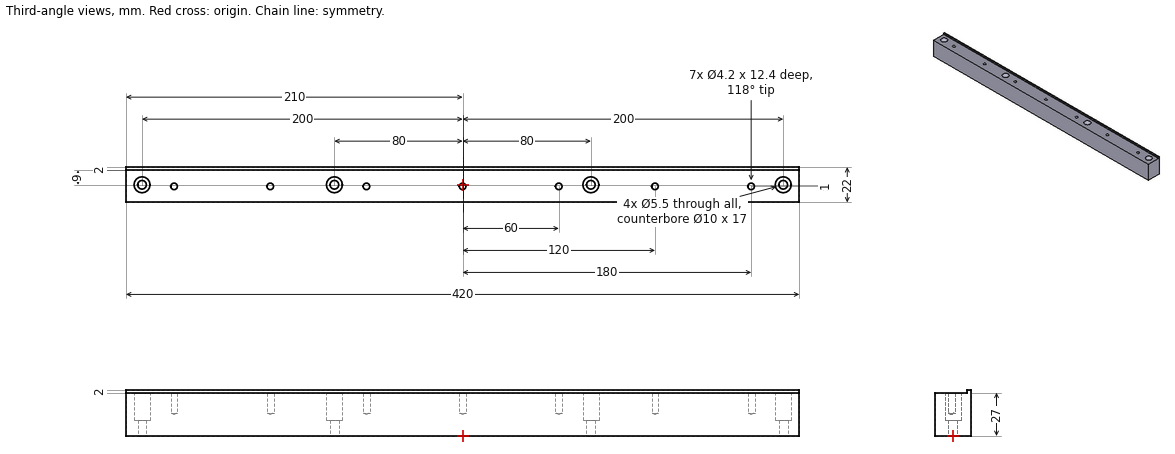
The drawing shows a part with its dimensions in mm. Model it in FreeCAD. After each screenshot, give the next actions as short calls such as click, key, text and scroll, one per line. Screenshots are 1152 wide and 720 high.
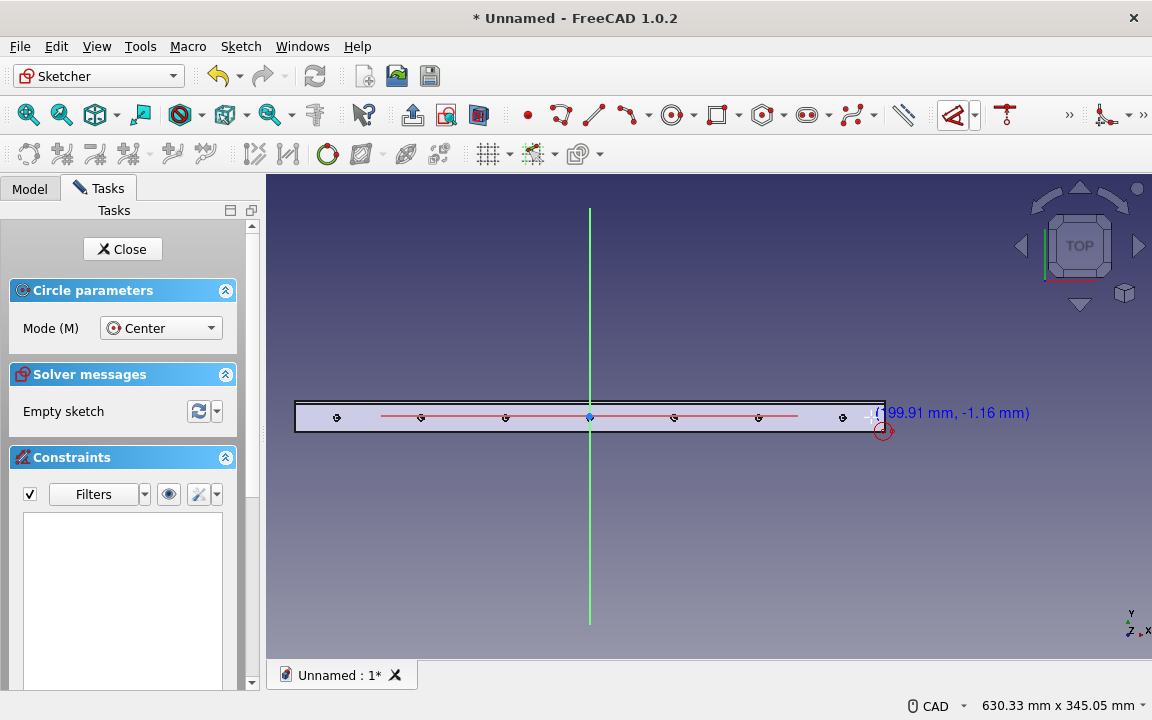
click(871, 417)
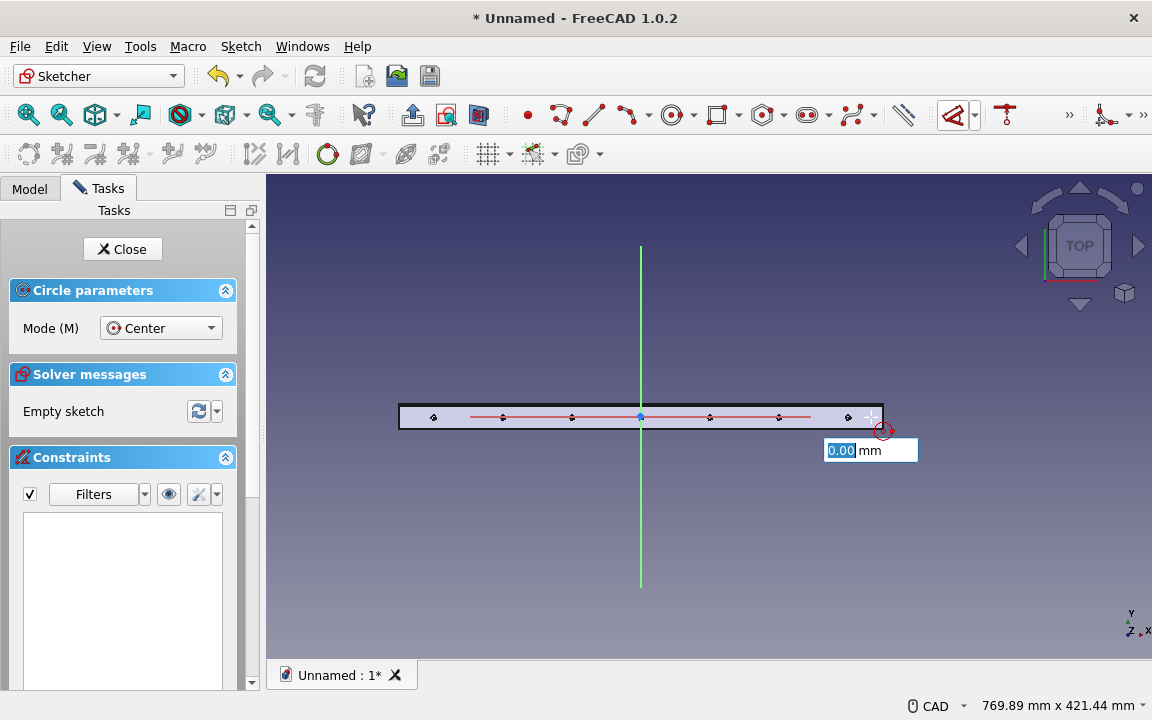
scroll(872, 414, up, 9)
move(870, 410)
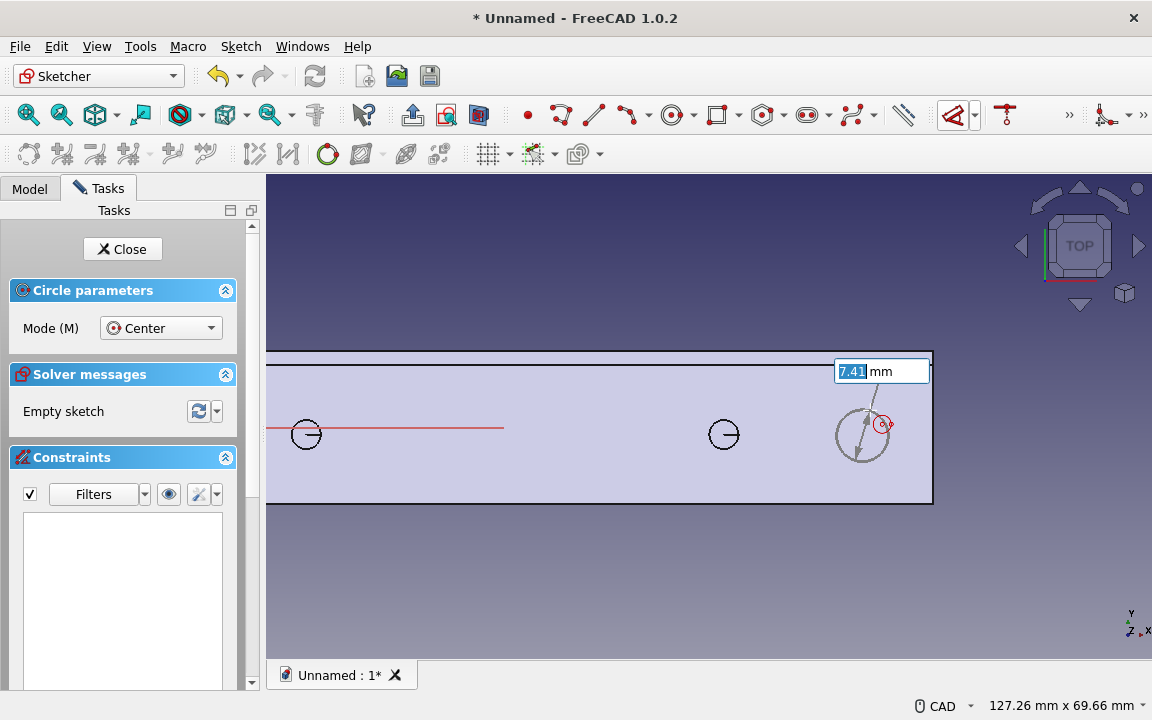
text(5.5)
key(Return)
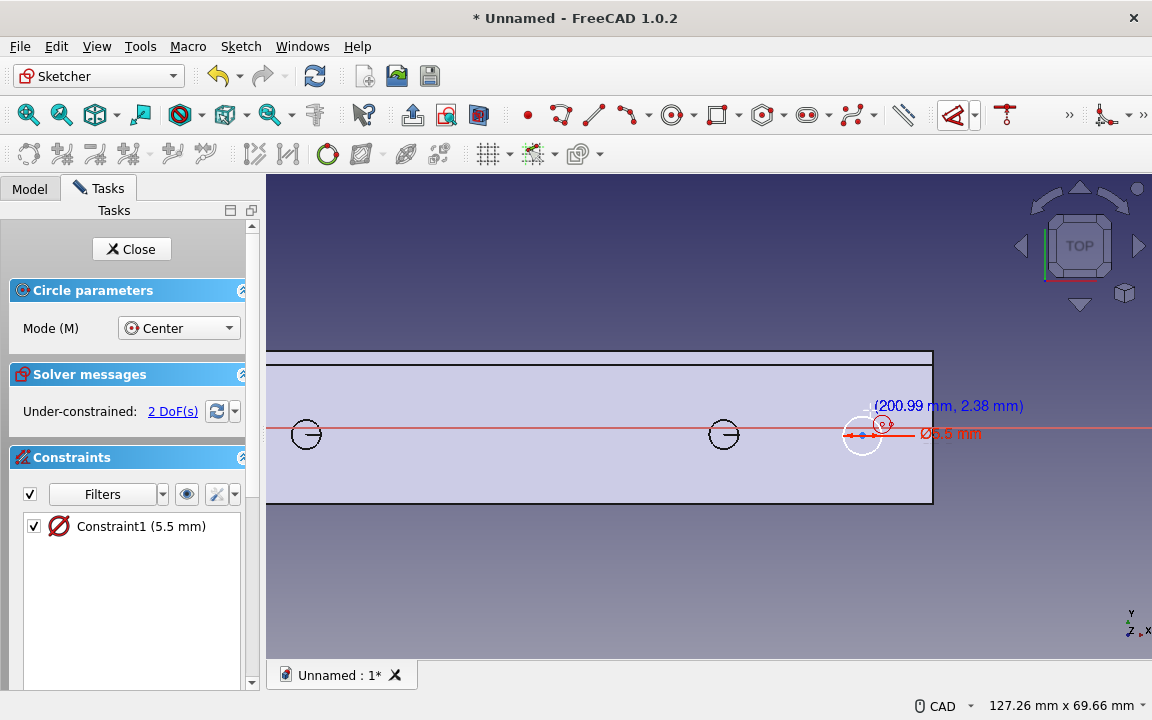
scroll(872, 414, down, 9)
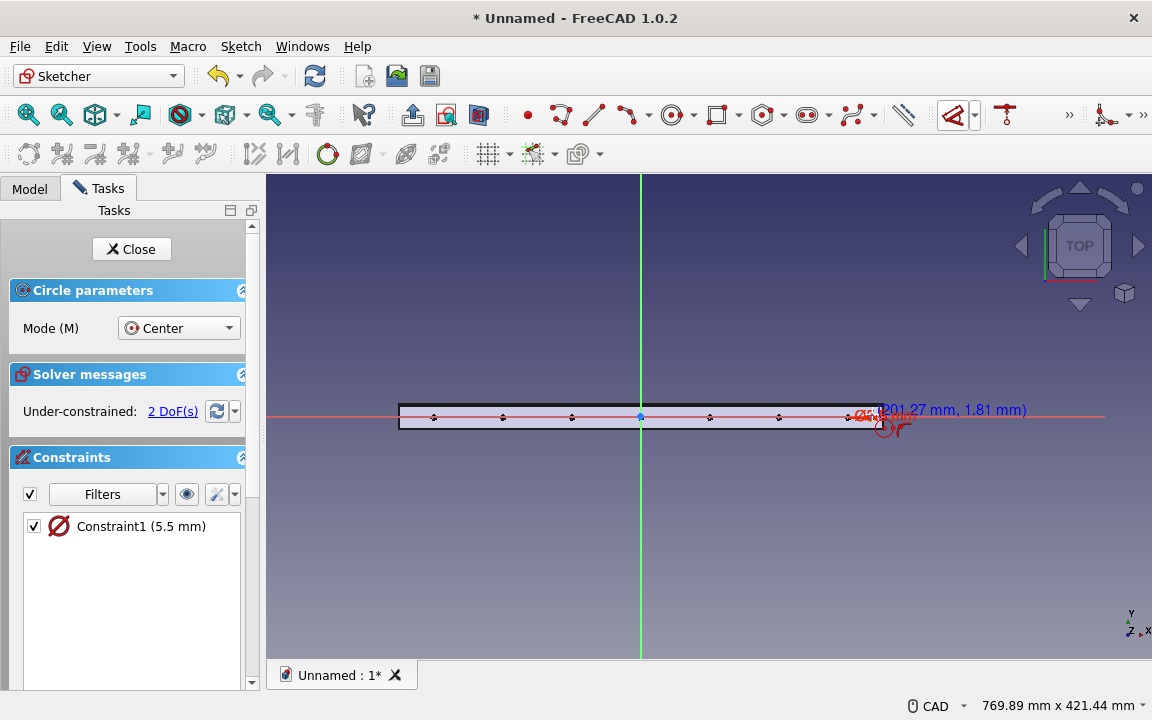
scroll(733, 417, up, 10)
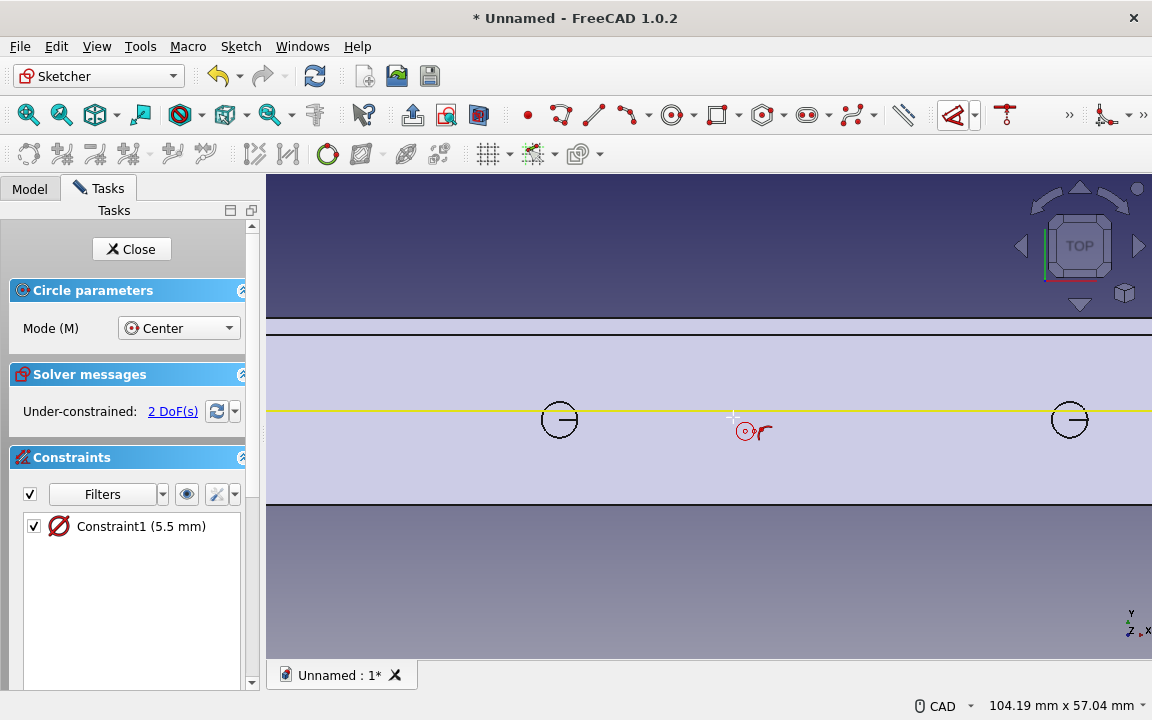
scroll(733, 417, down, 10)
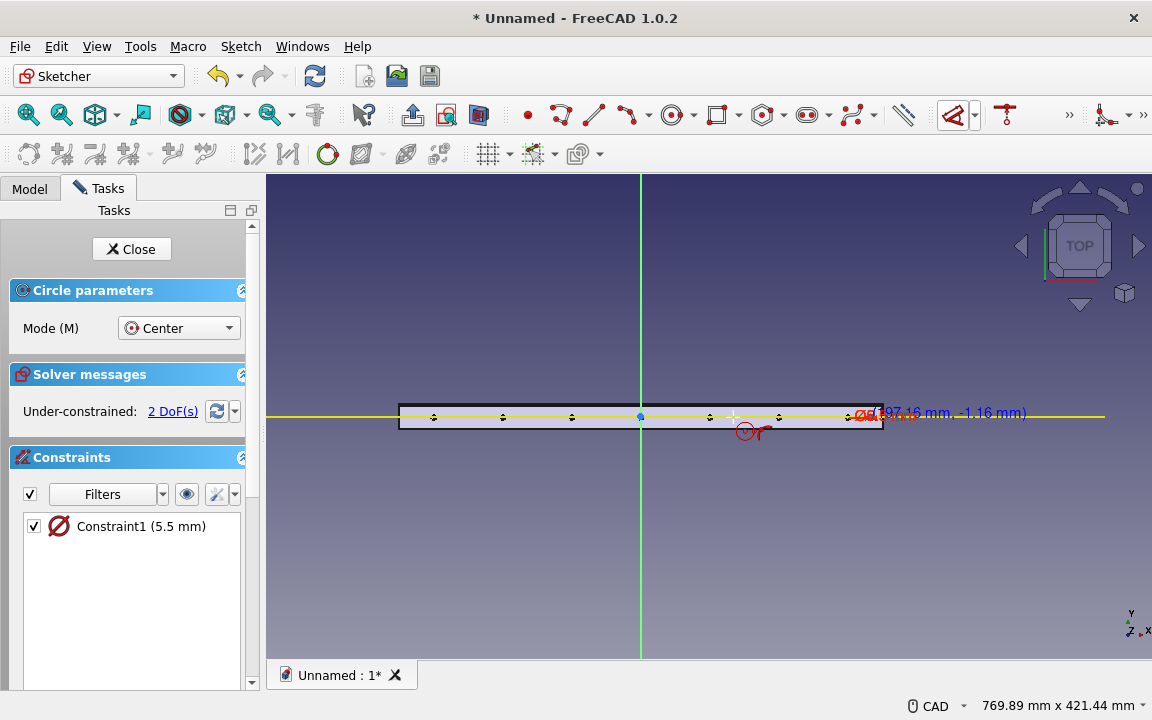
click(733, 417)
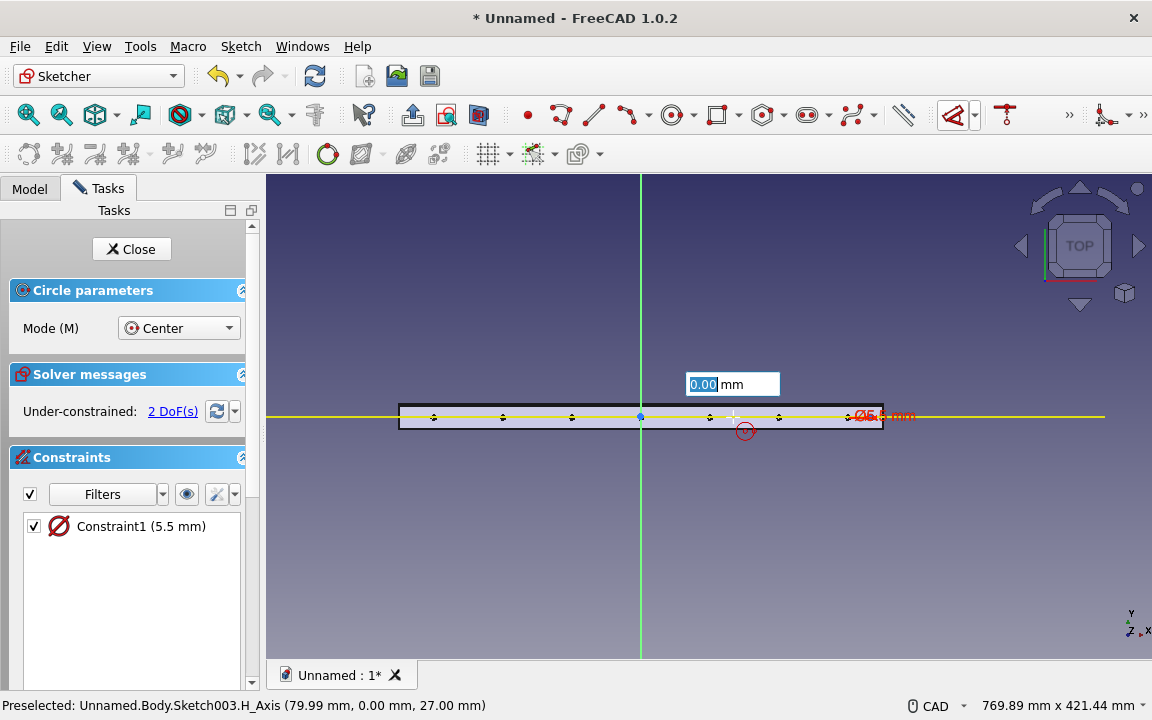
scroll(734, 414, up, 9)
move(732, 410)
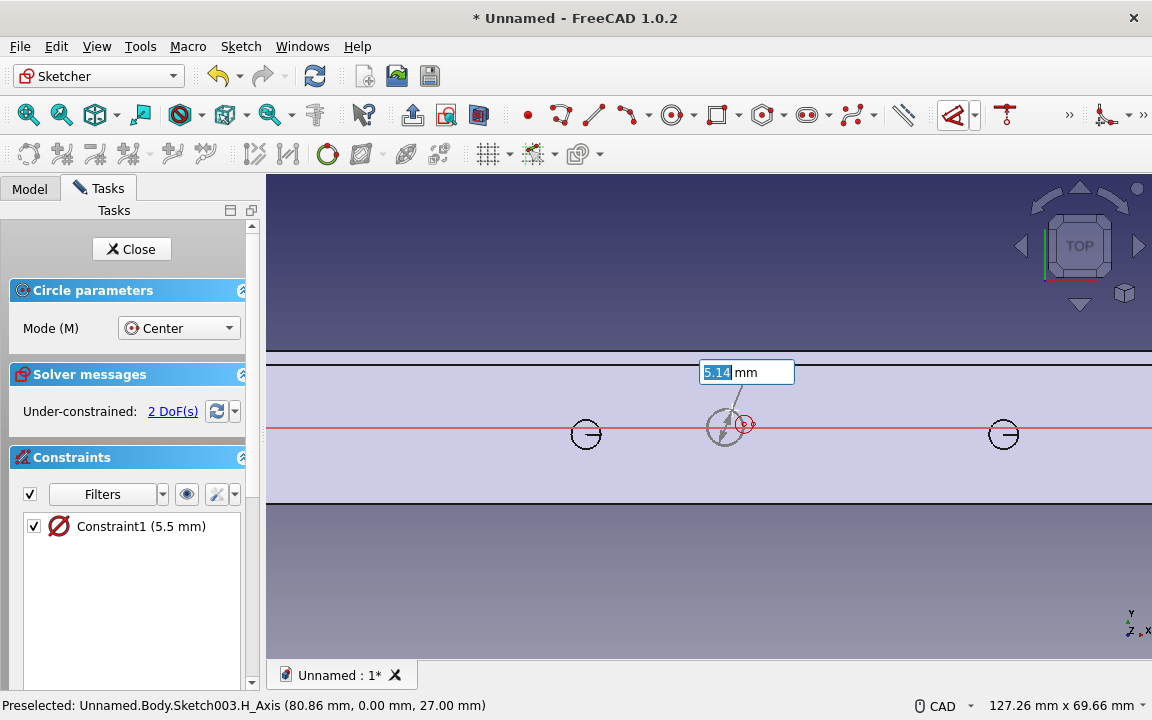
text(5.5)
key(Return)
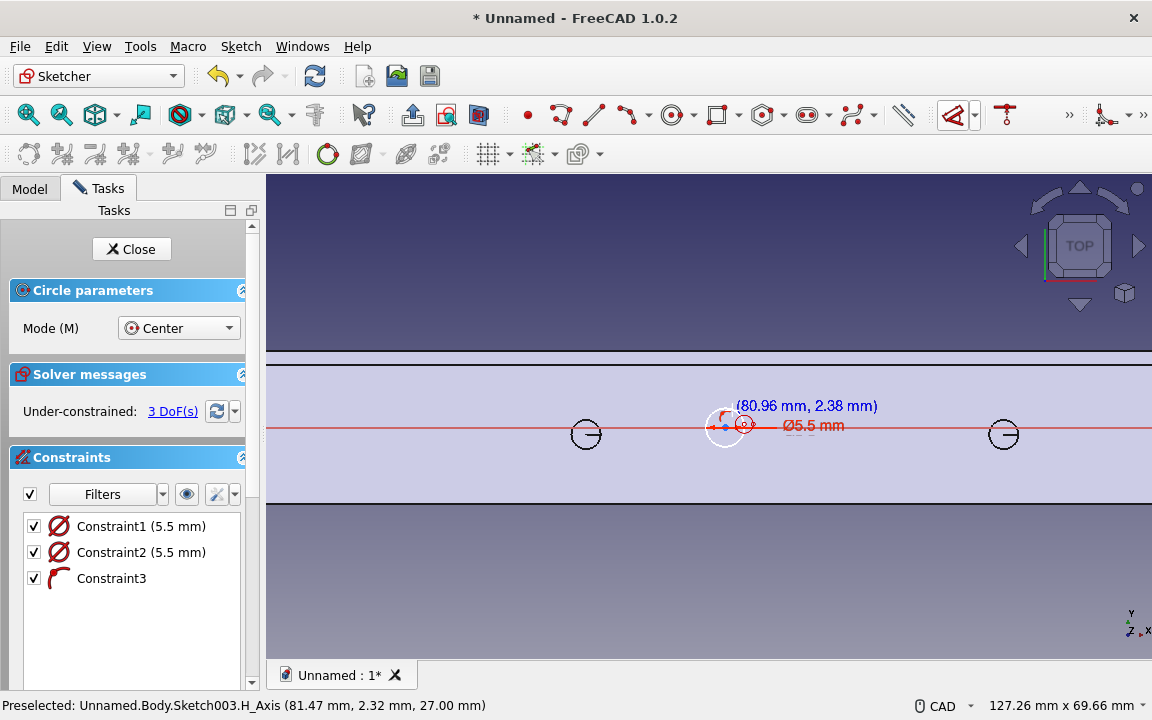
scroll(734, 414, down, 9)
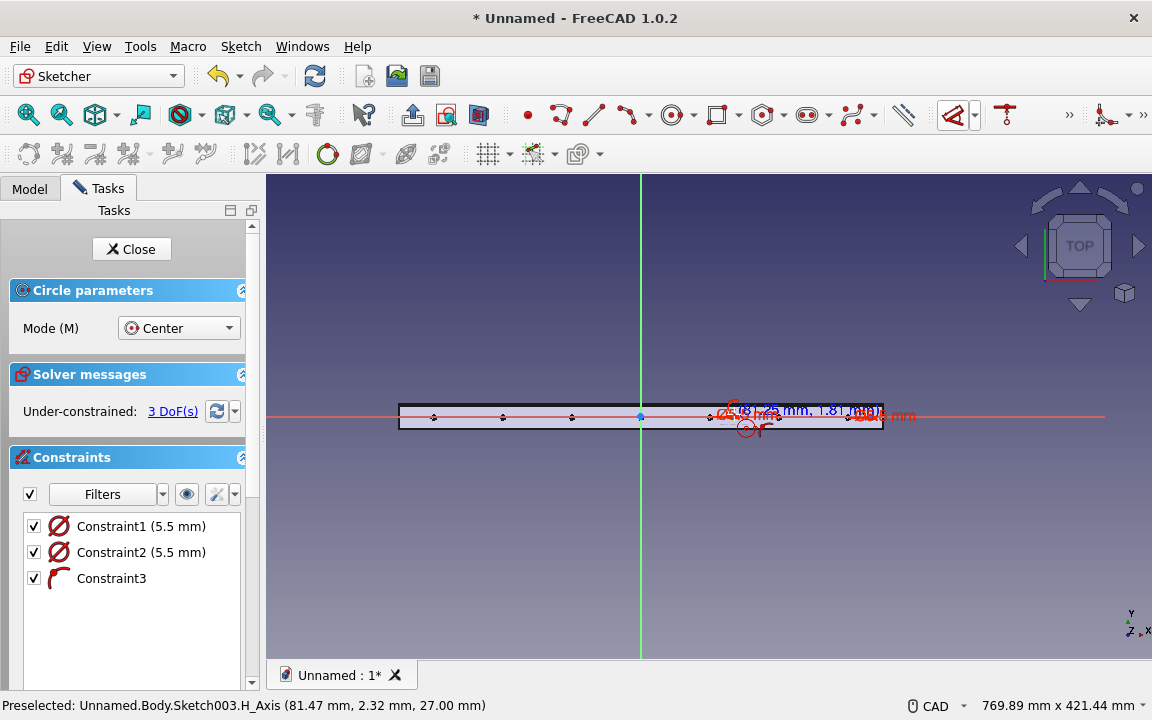
scroll(549, 417, up, 10)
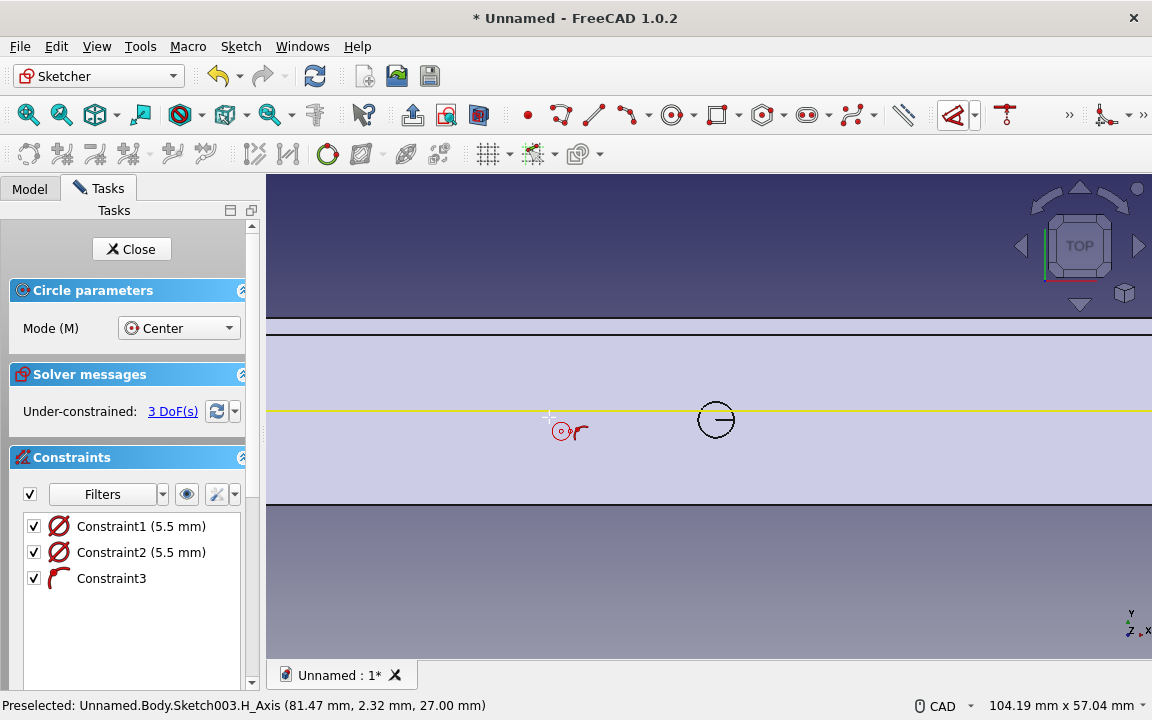
scroll(549, 417, down, 10)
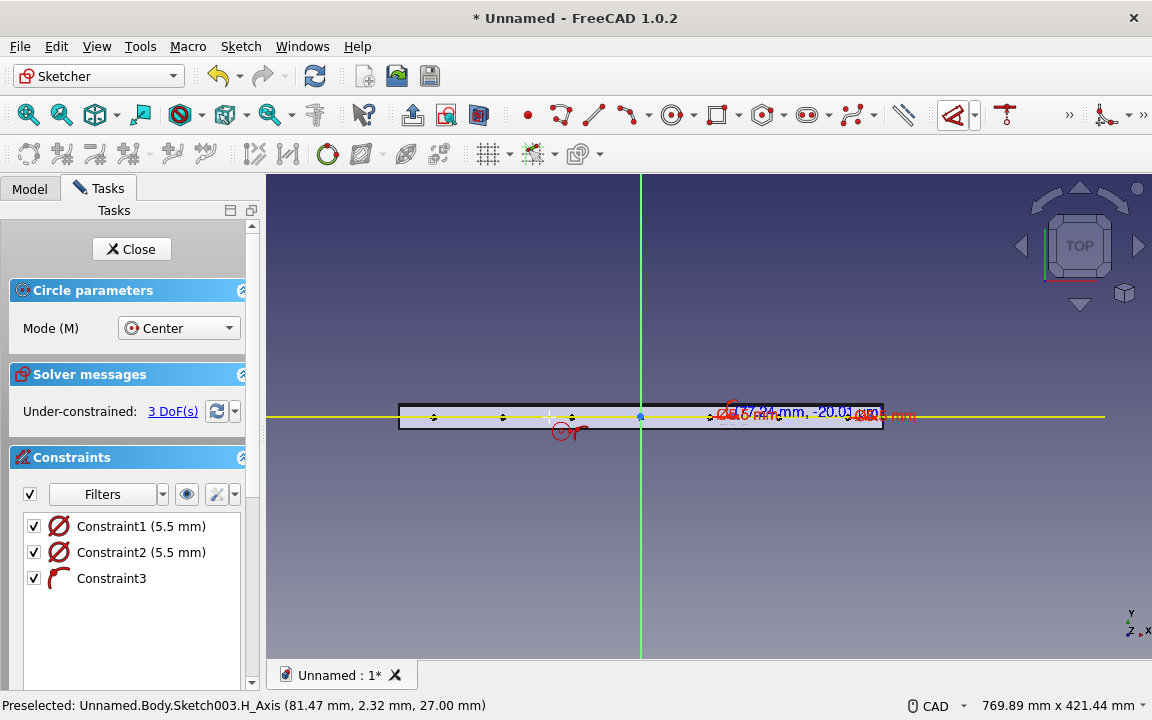
click(549, 417)